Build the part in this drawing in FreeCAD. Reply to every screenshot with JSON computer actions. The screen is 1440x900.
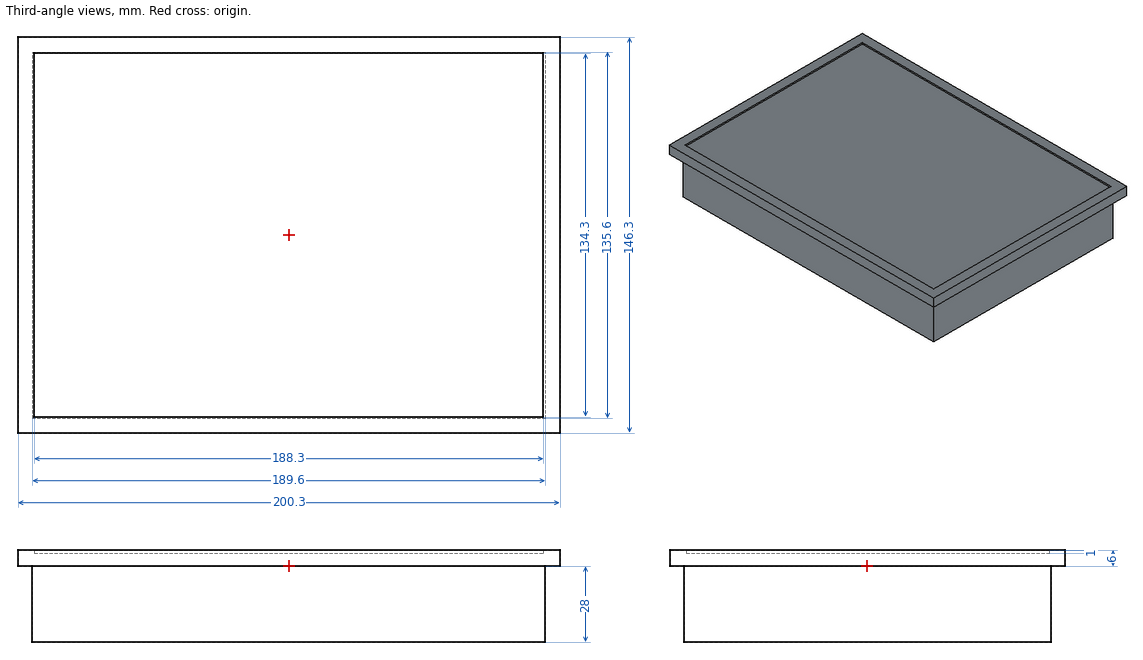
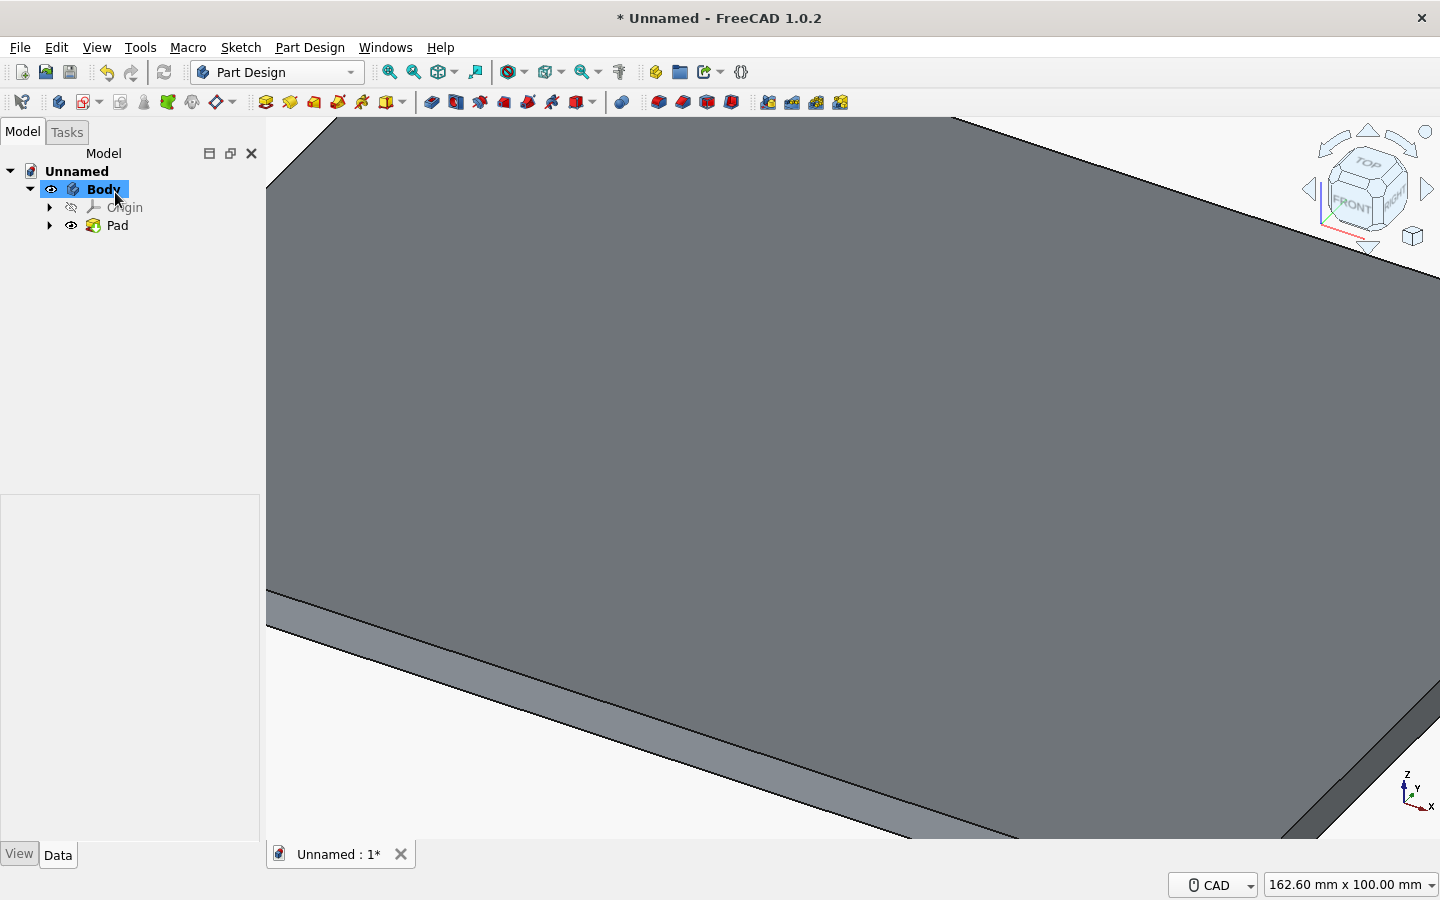
{"action": "left_click", "coordinate": [390, 72]}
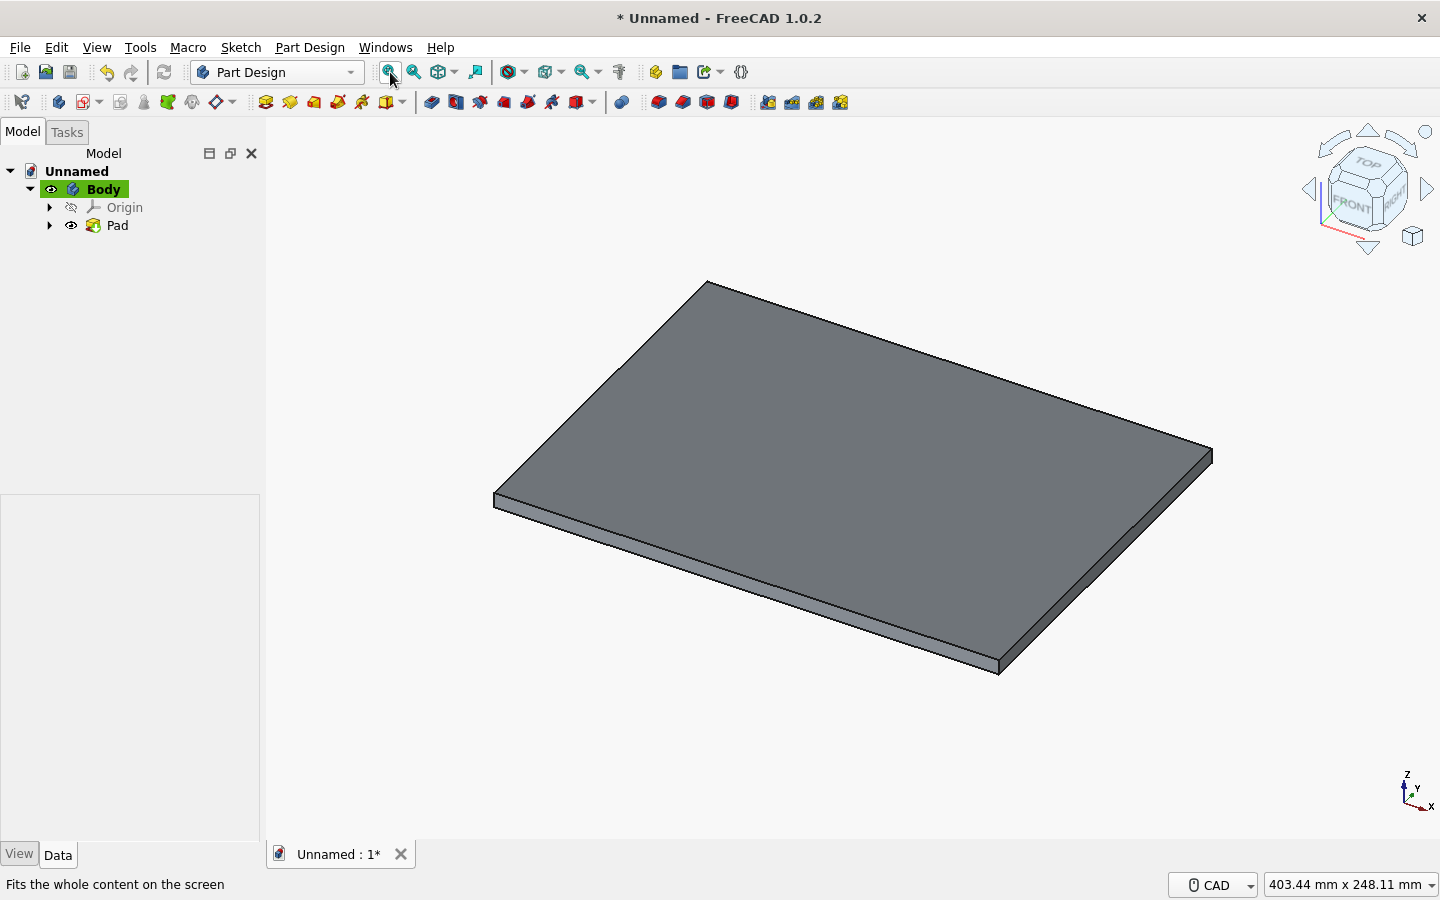
{"action": "left_click", "coordinate": [84, 102]}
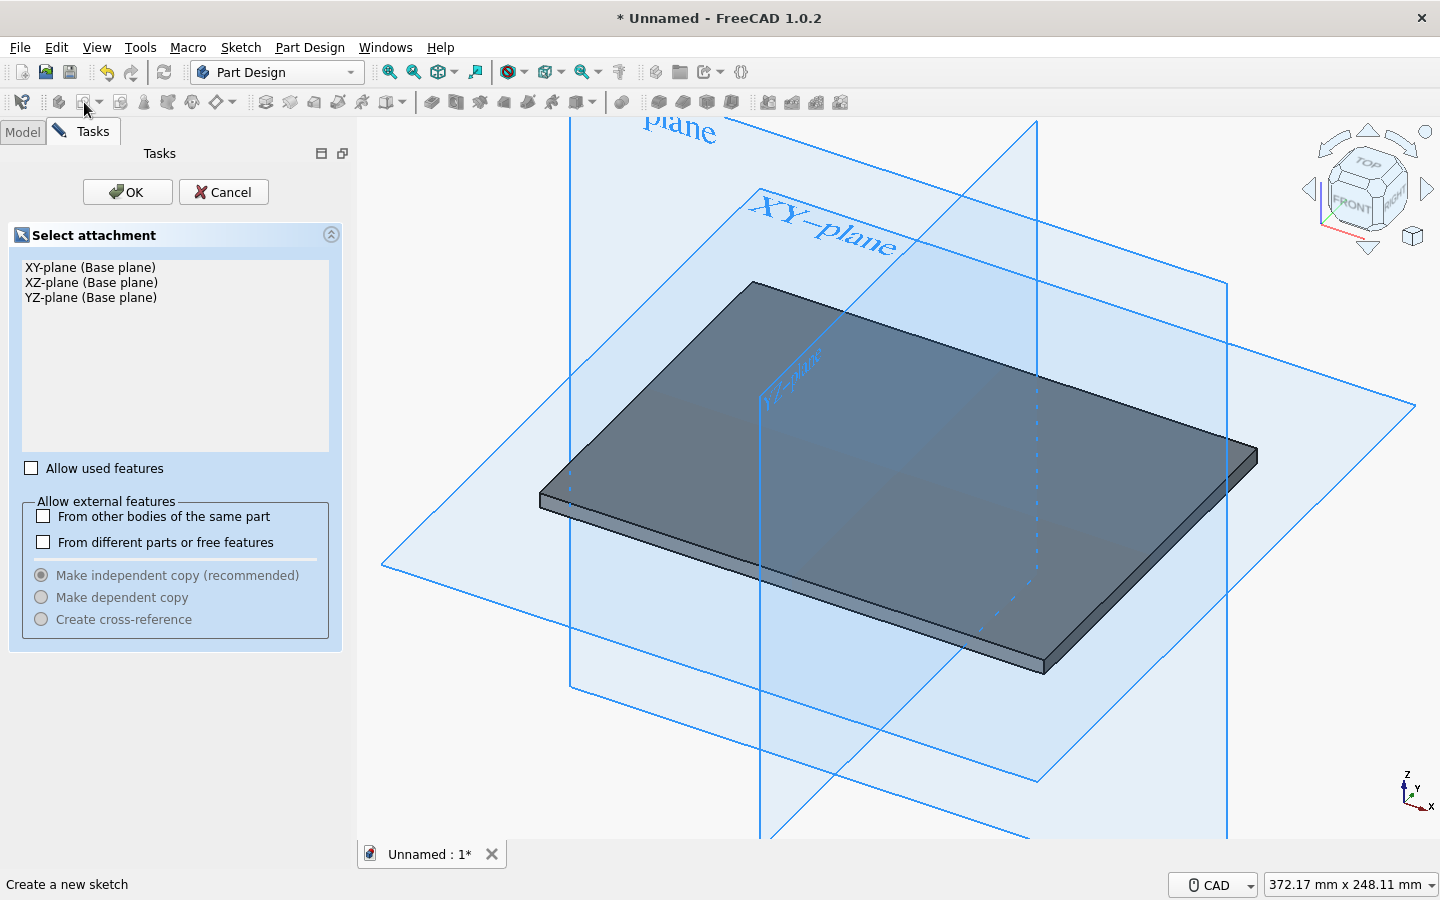
{"action": "left_click", "coordinate": [82, 268]}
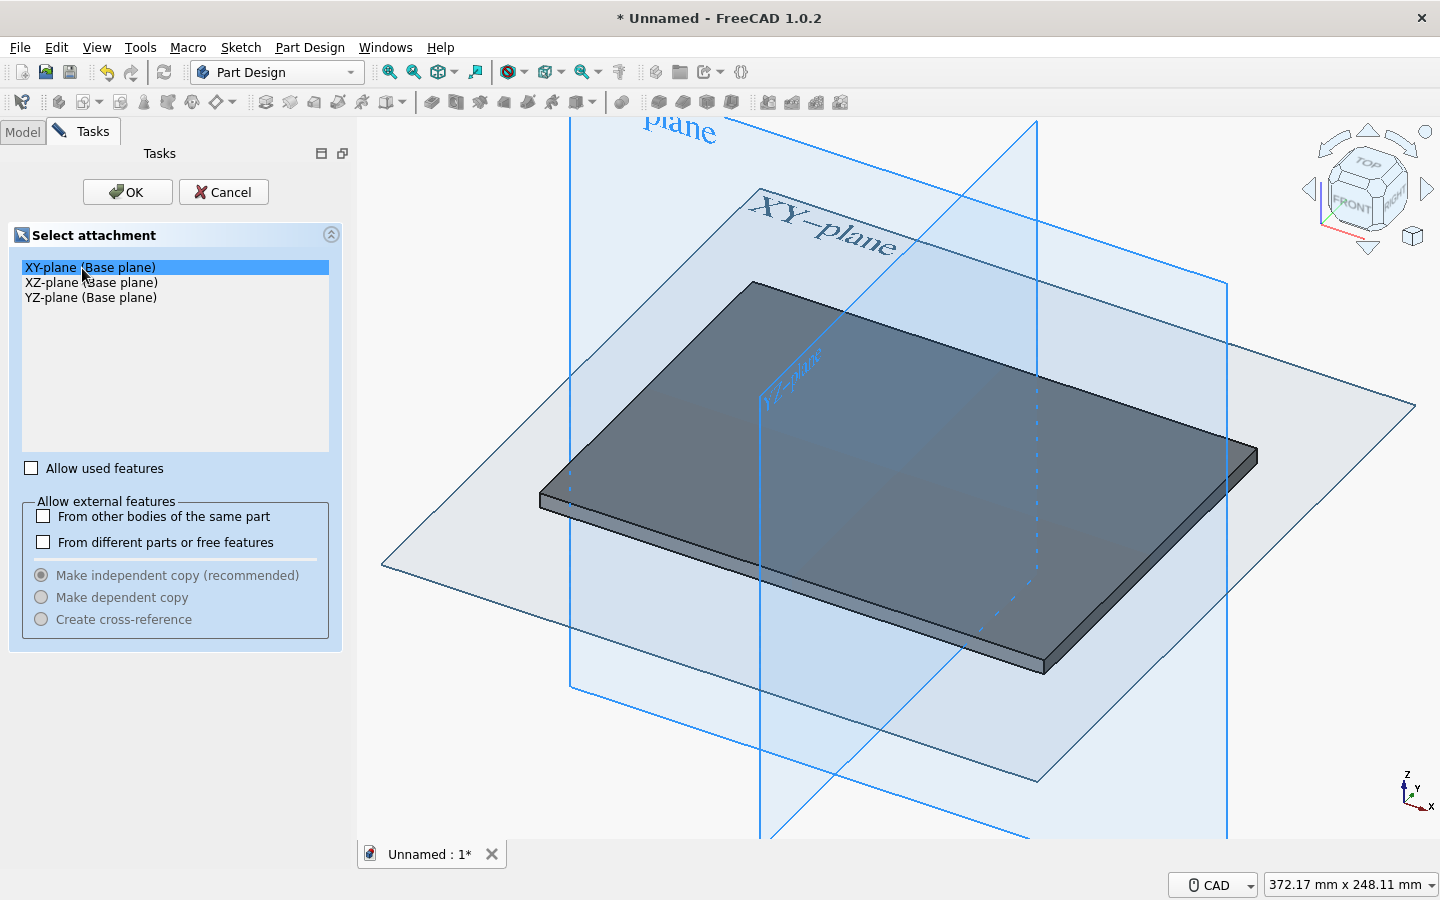
{"action": "left_click", "coordinate": [128, 192]}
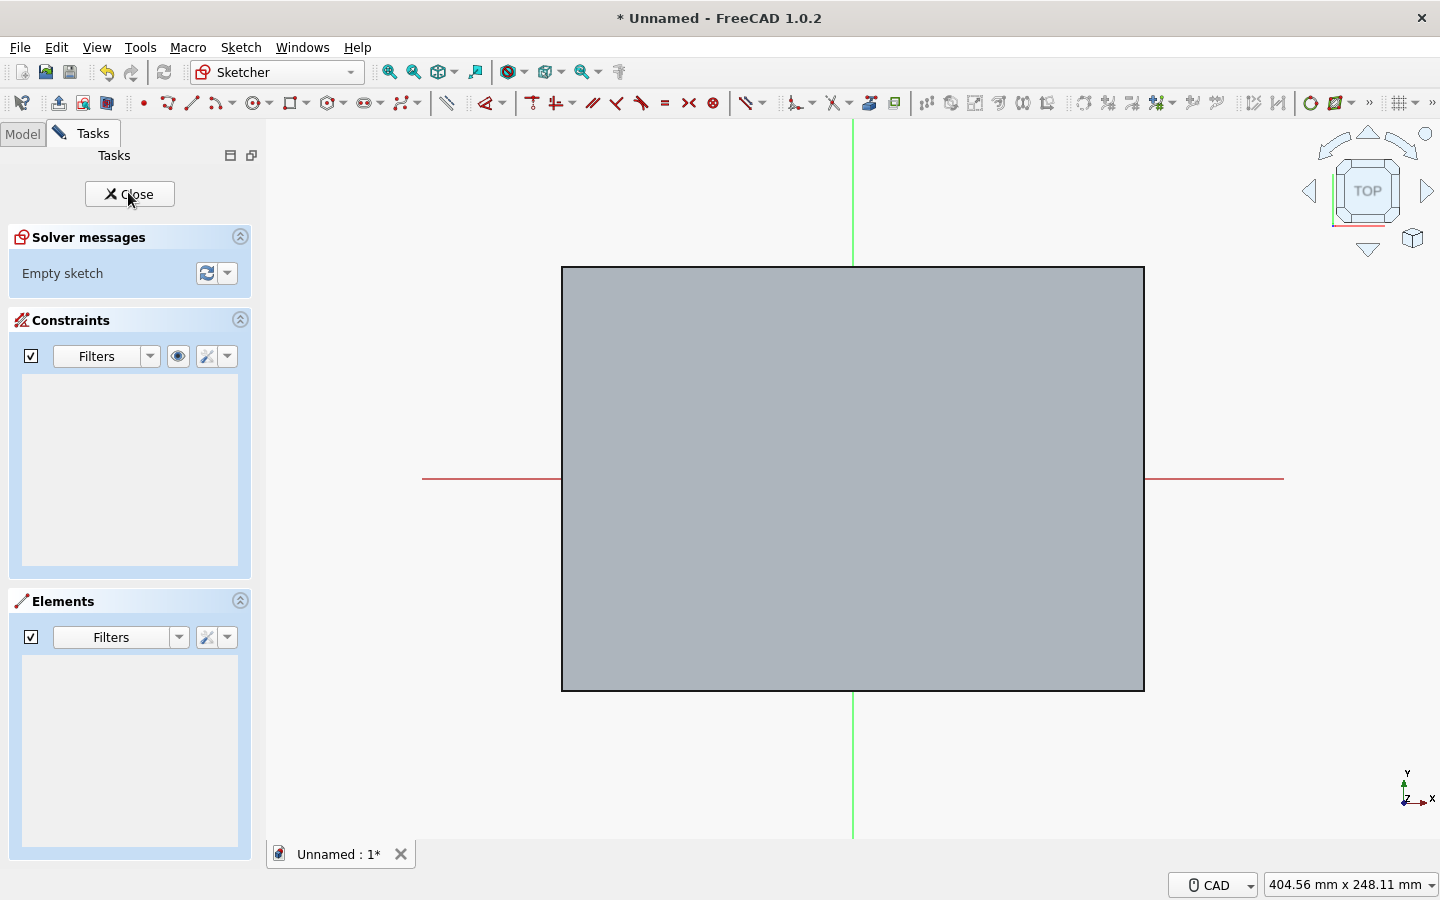
{"action": "left_click", "coordinate": [108, 104]}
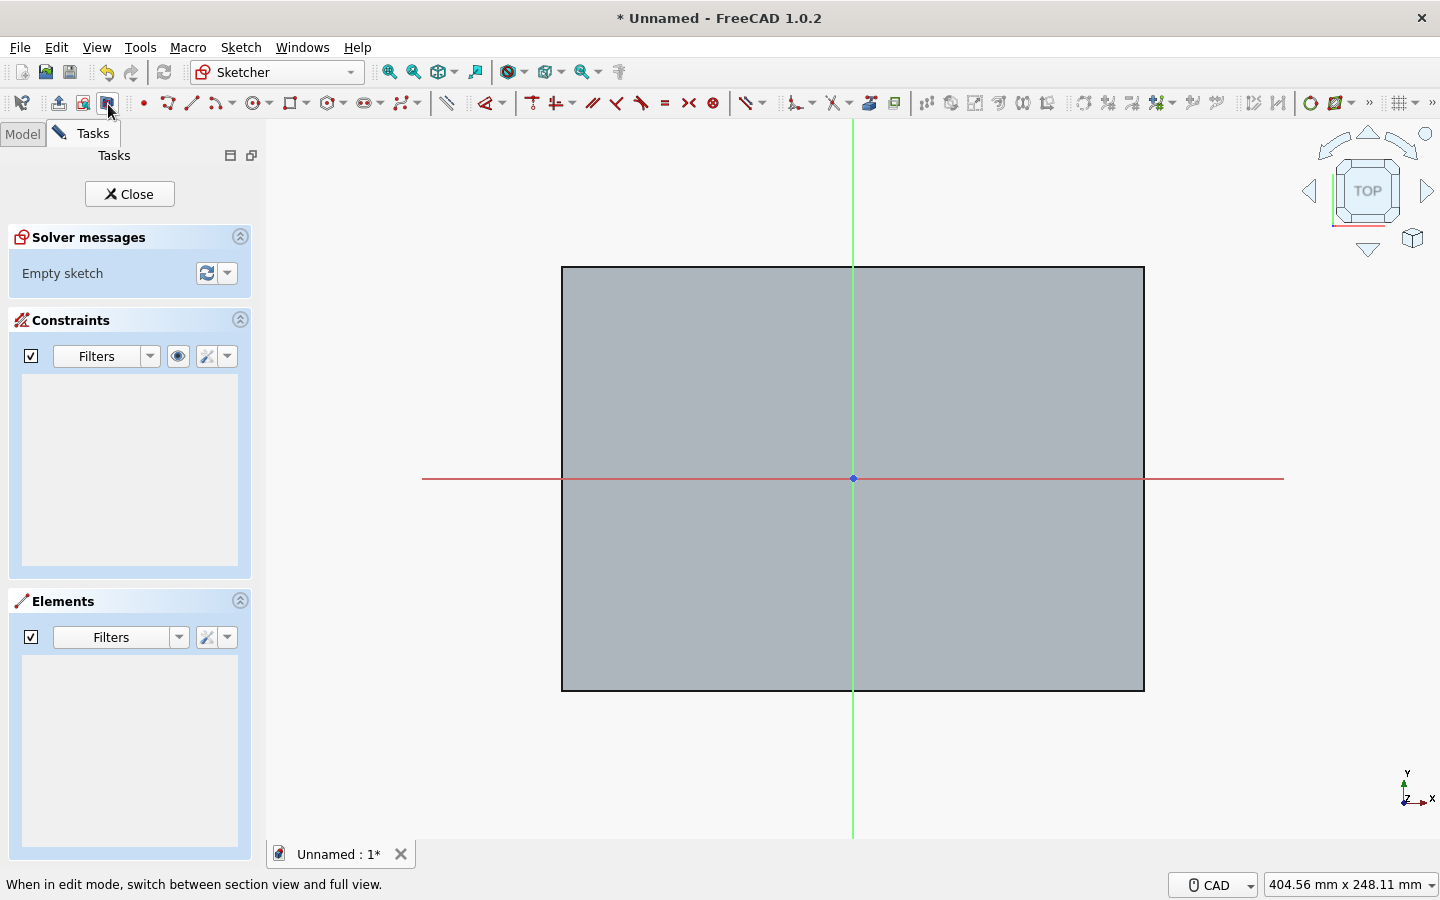
{"action": "key", "text": "g v"}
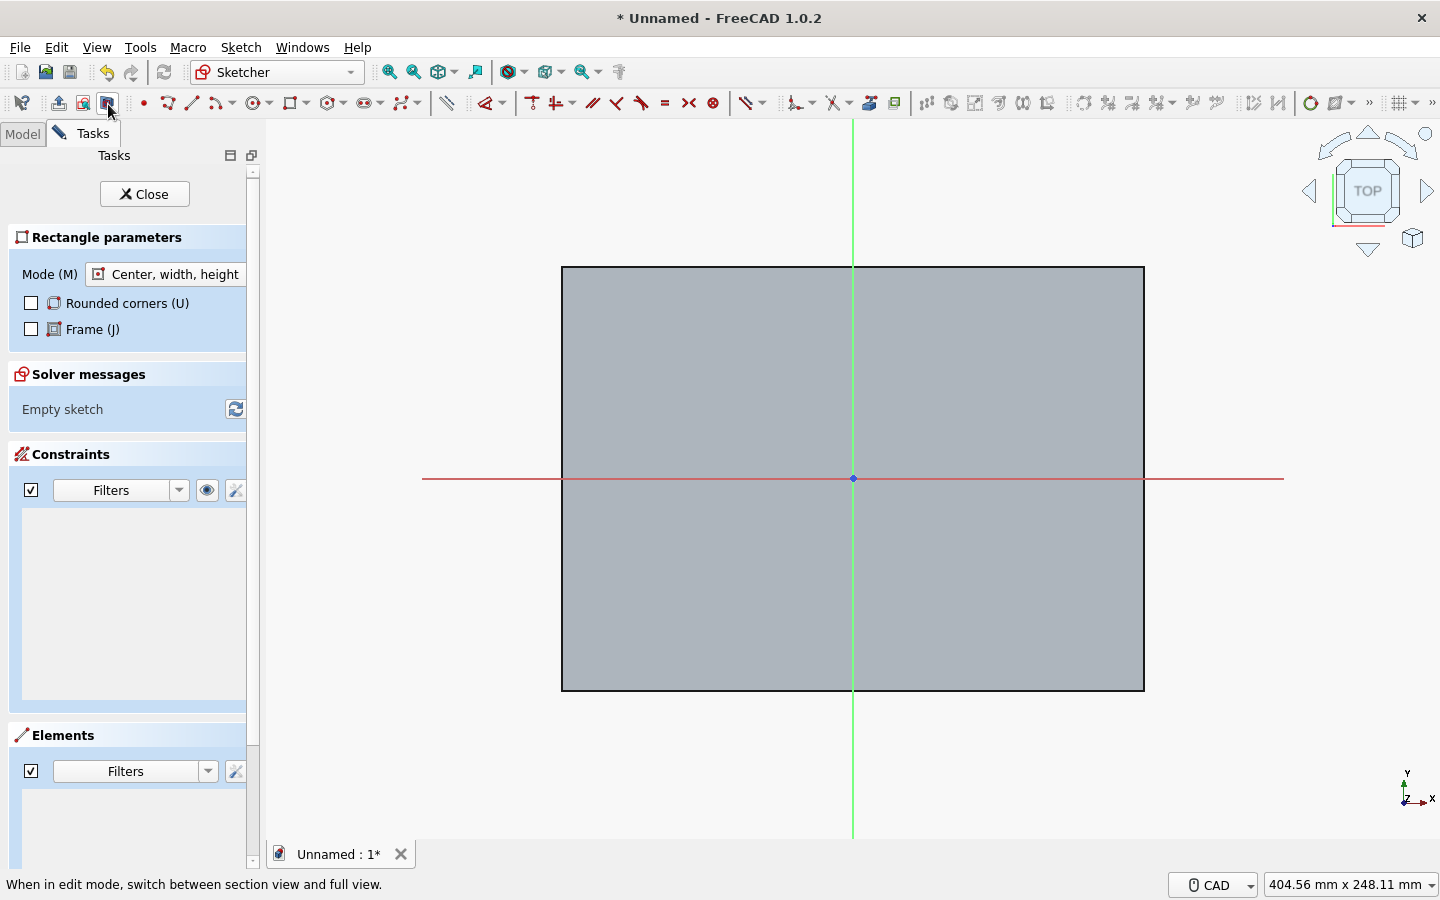
{"action": "left_click", "coordinate": [853, 479]}
{"action": "left_click", "coordinate": [1128, 282]}
{"action": "key", "text": "Escape"}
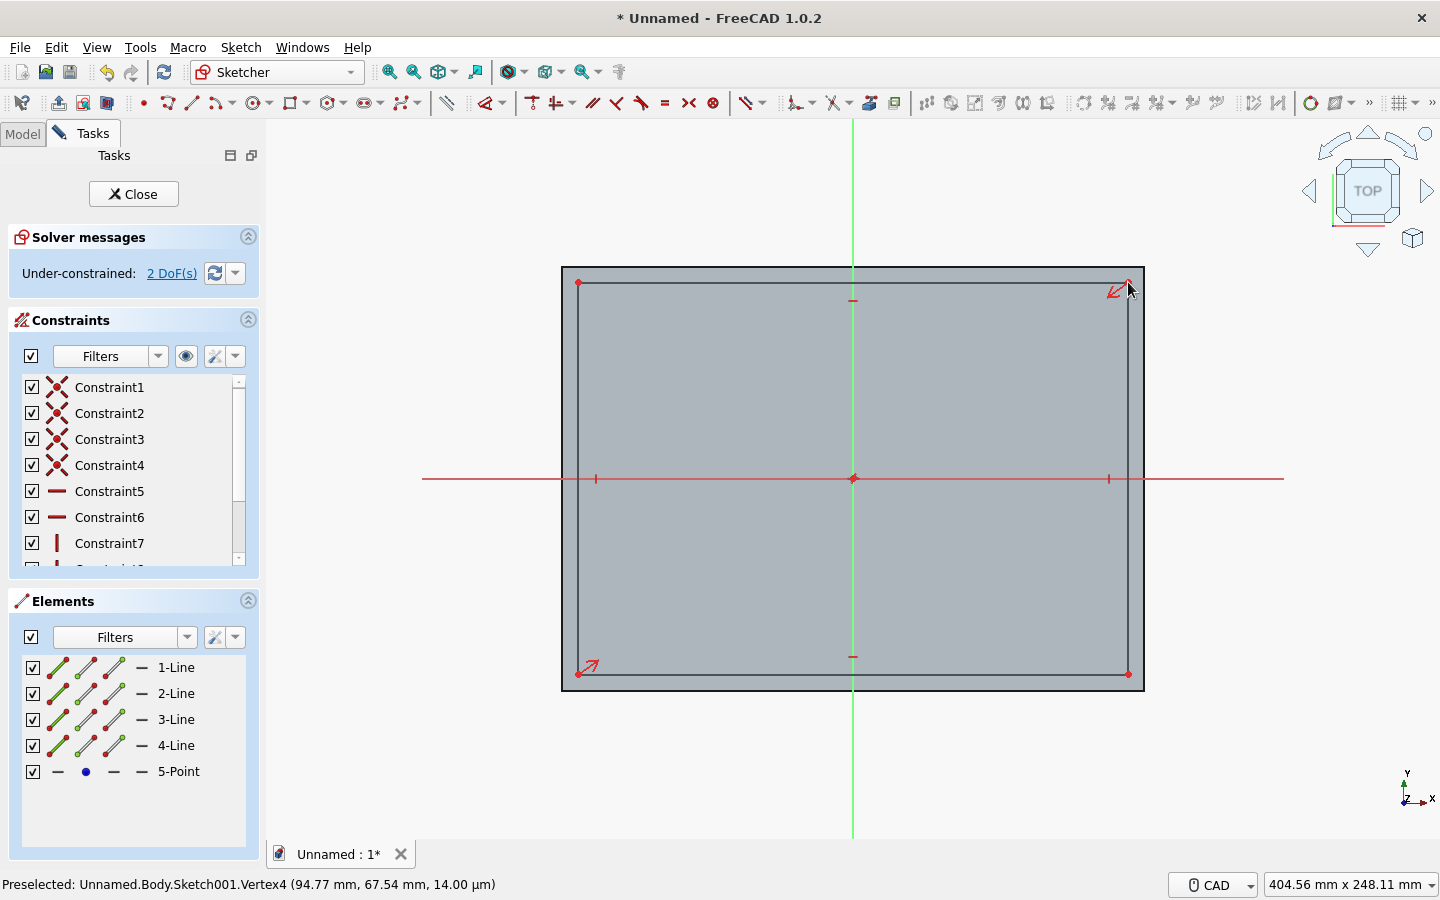
{"action": "left_click", "coordinate": [486, 104]}